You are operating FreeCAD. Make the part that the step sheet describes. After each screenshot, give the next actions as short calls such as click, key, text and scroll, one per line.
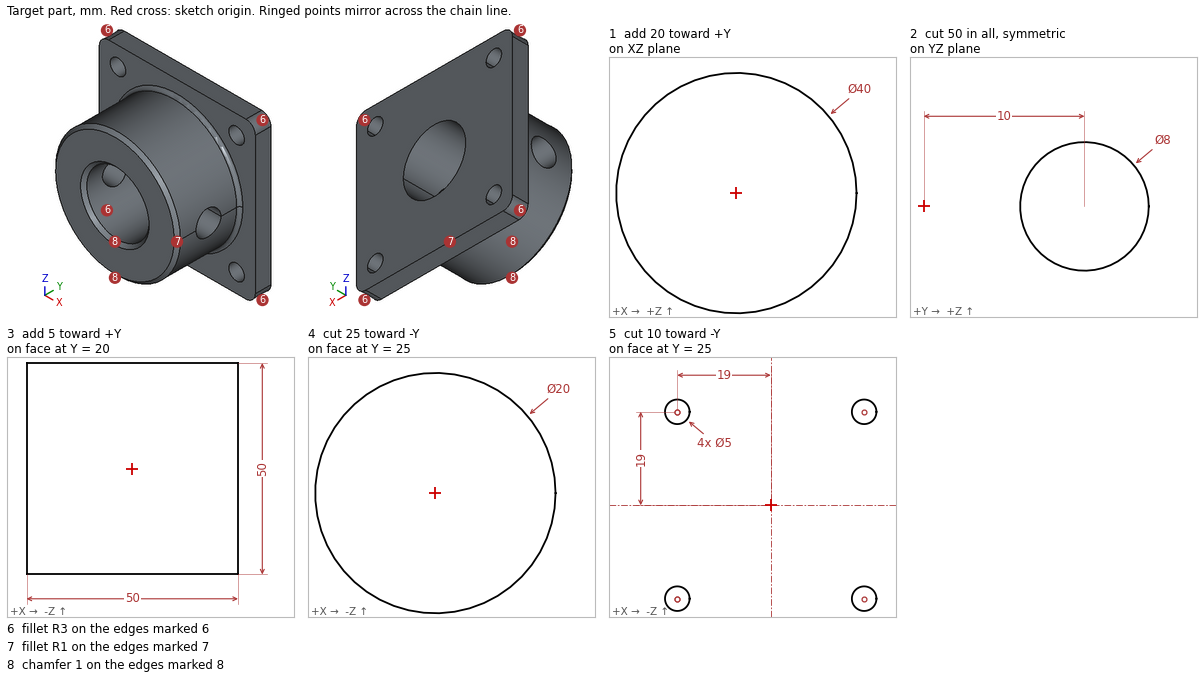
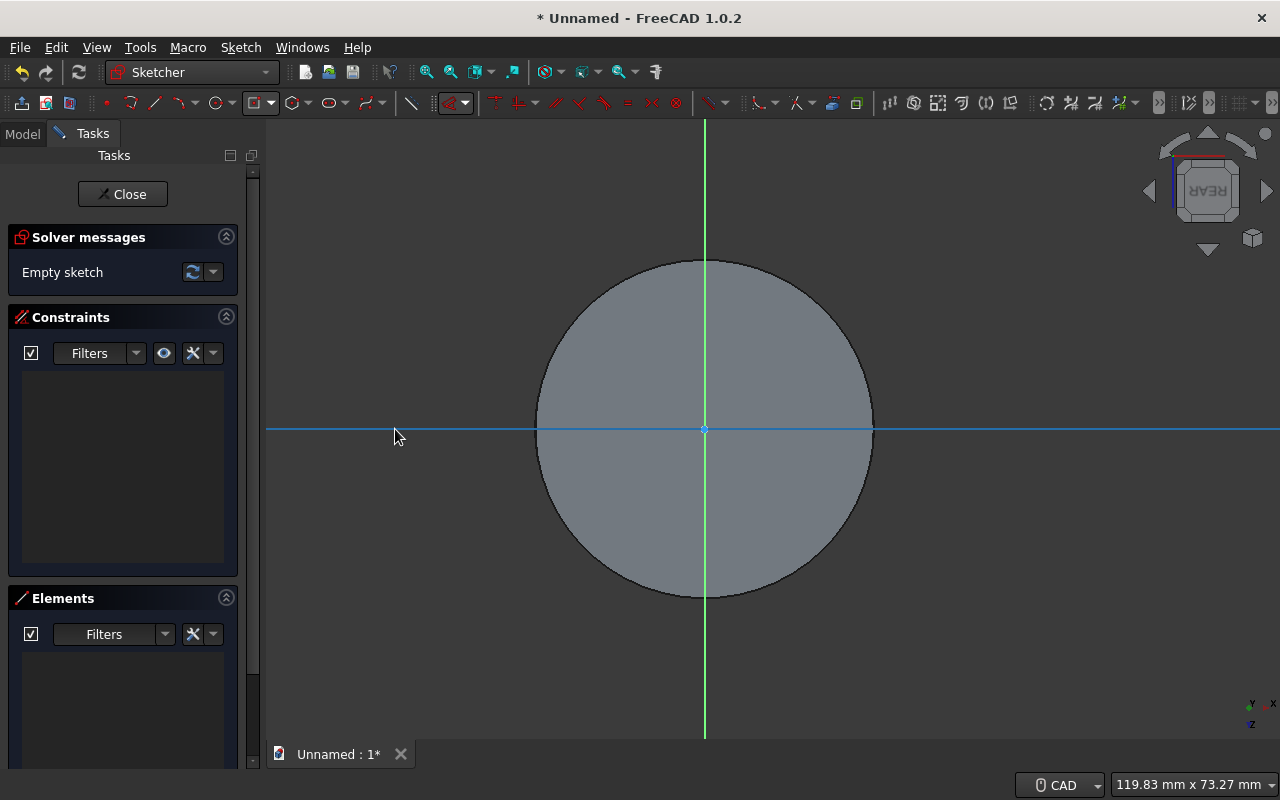
click(254, 104)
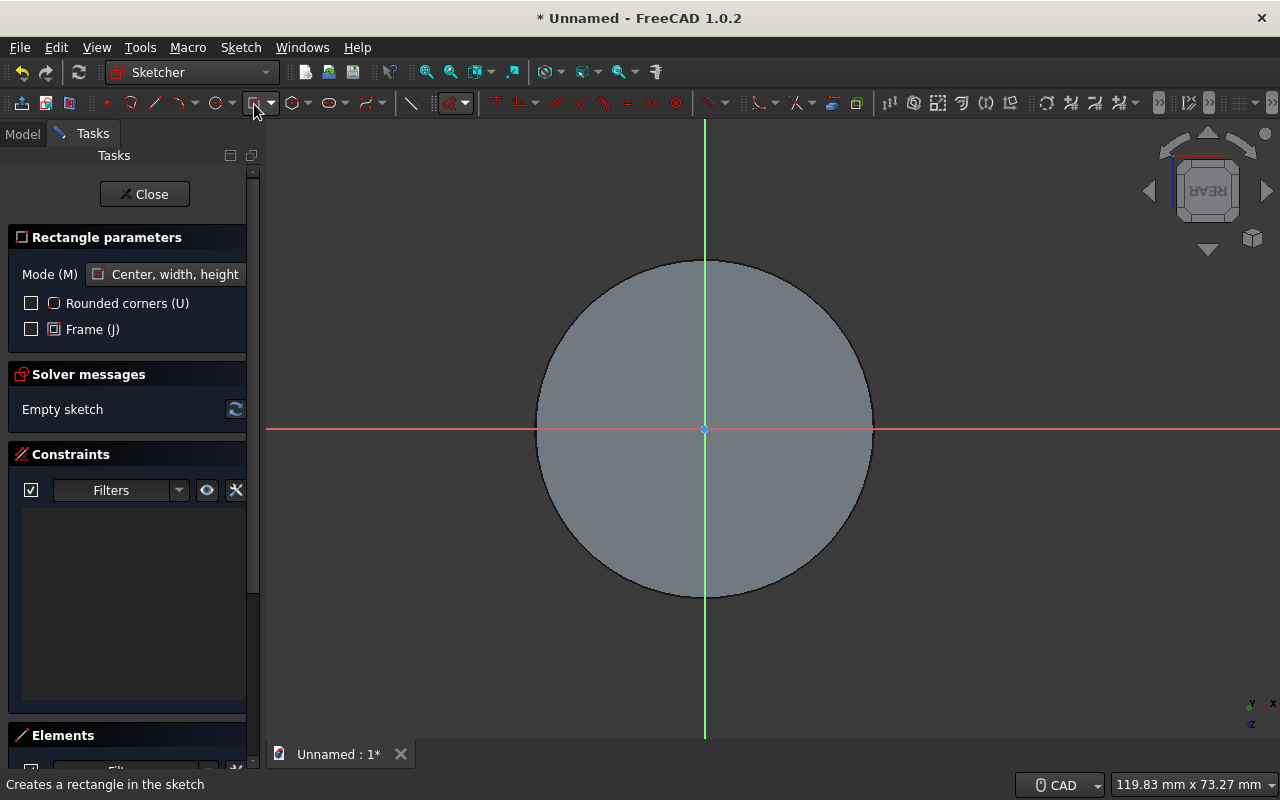
click(705, 429)
click(916, 218)
key(Escape)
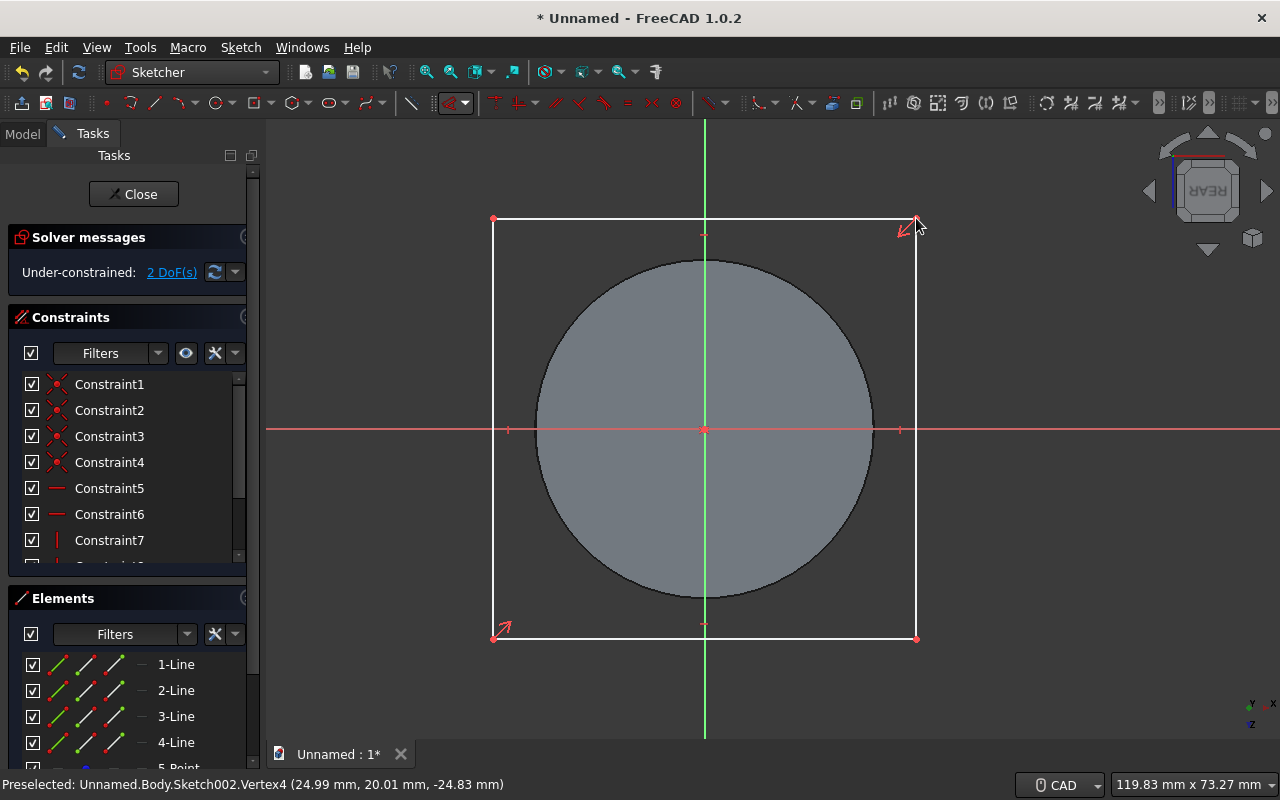
click(620, 639)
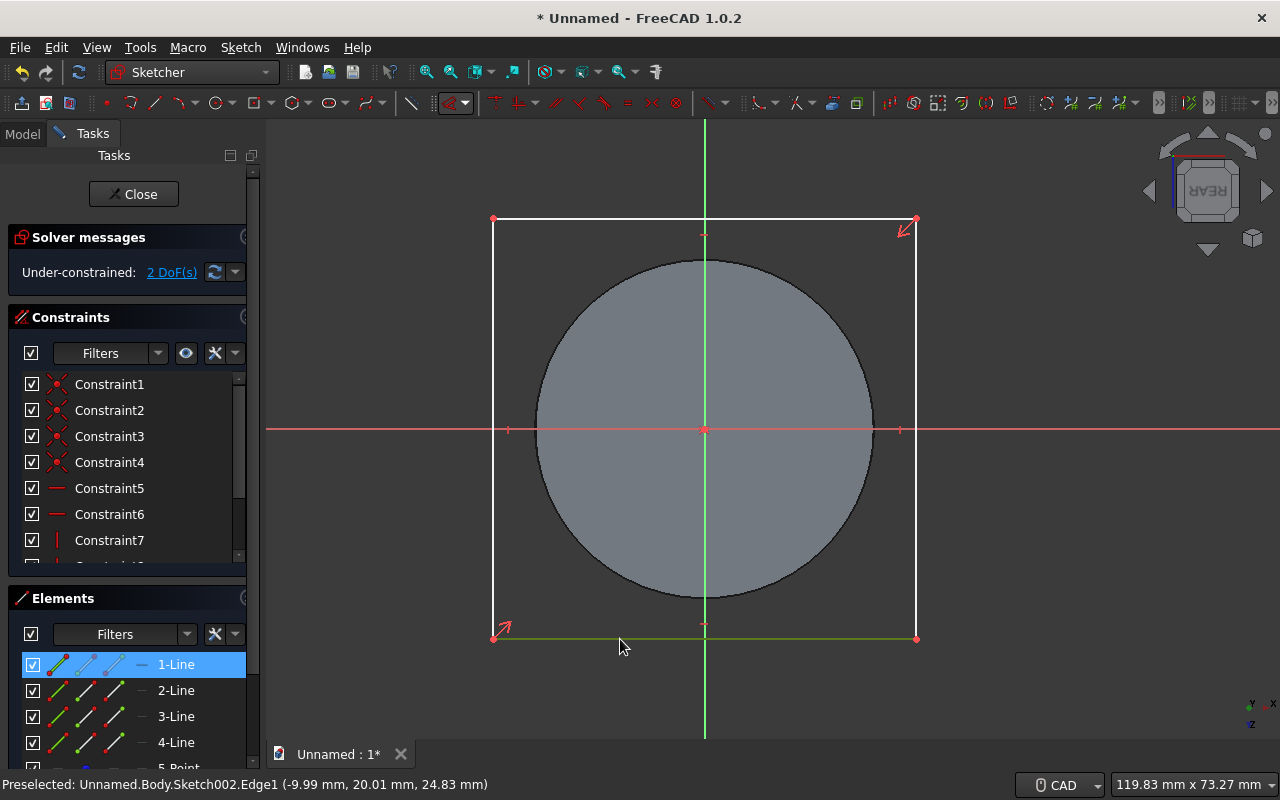
key(l)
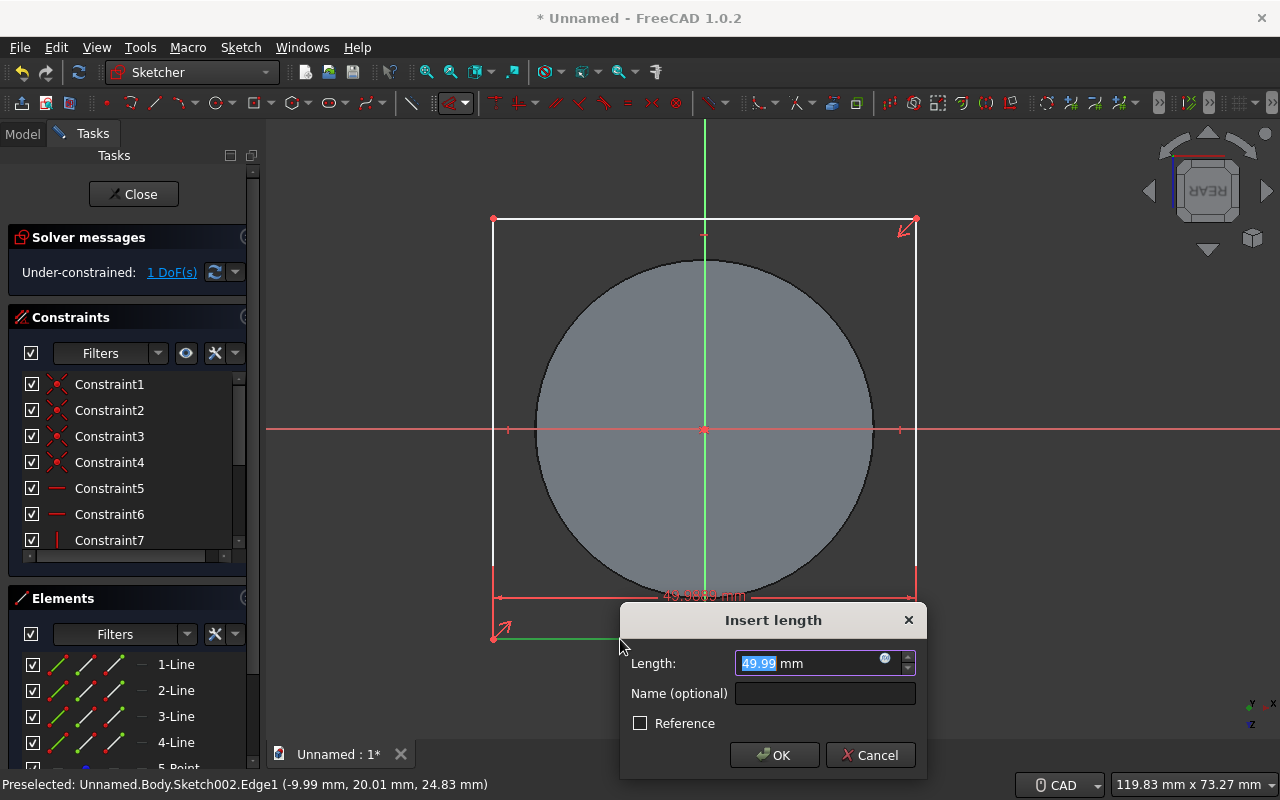
text(50)
key(Return)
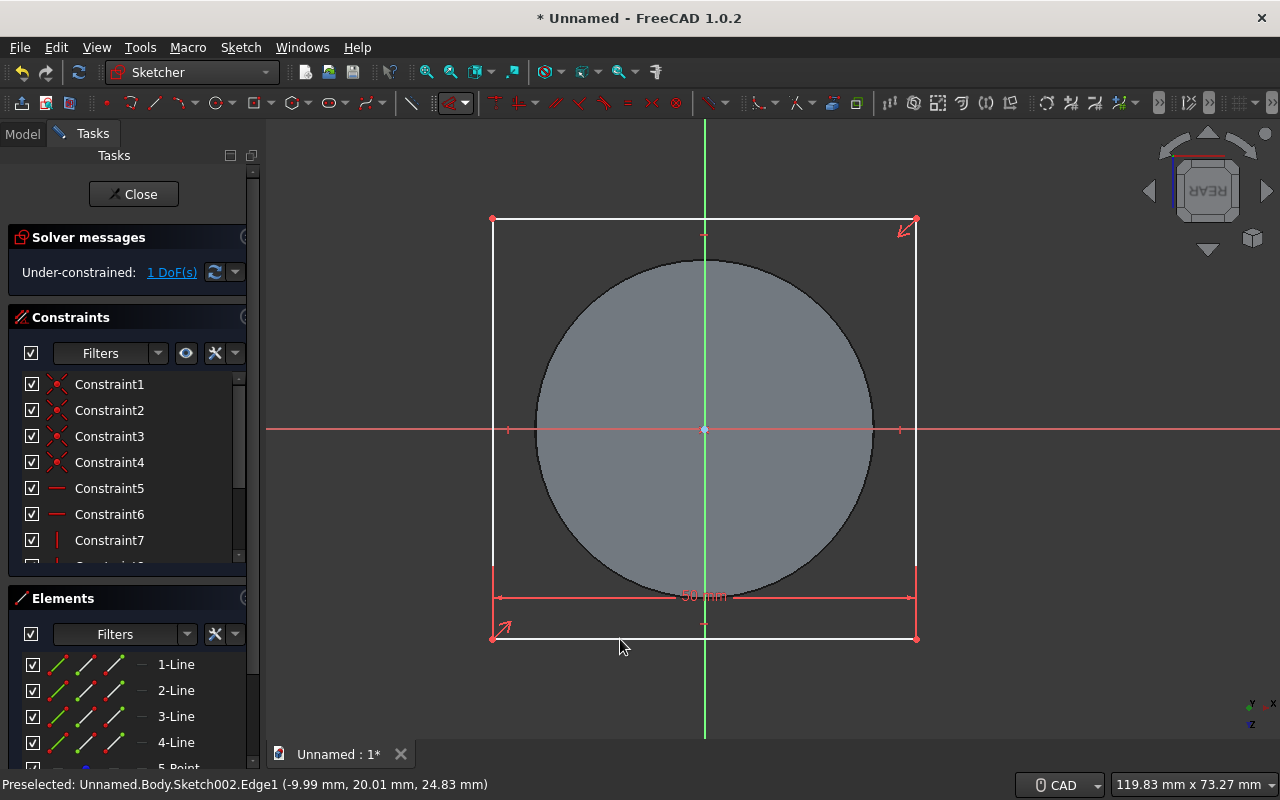
click(916, 513)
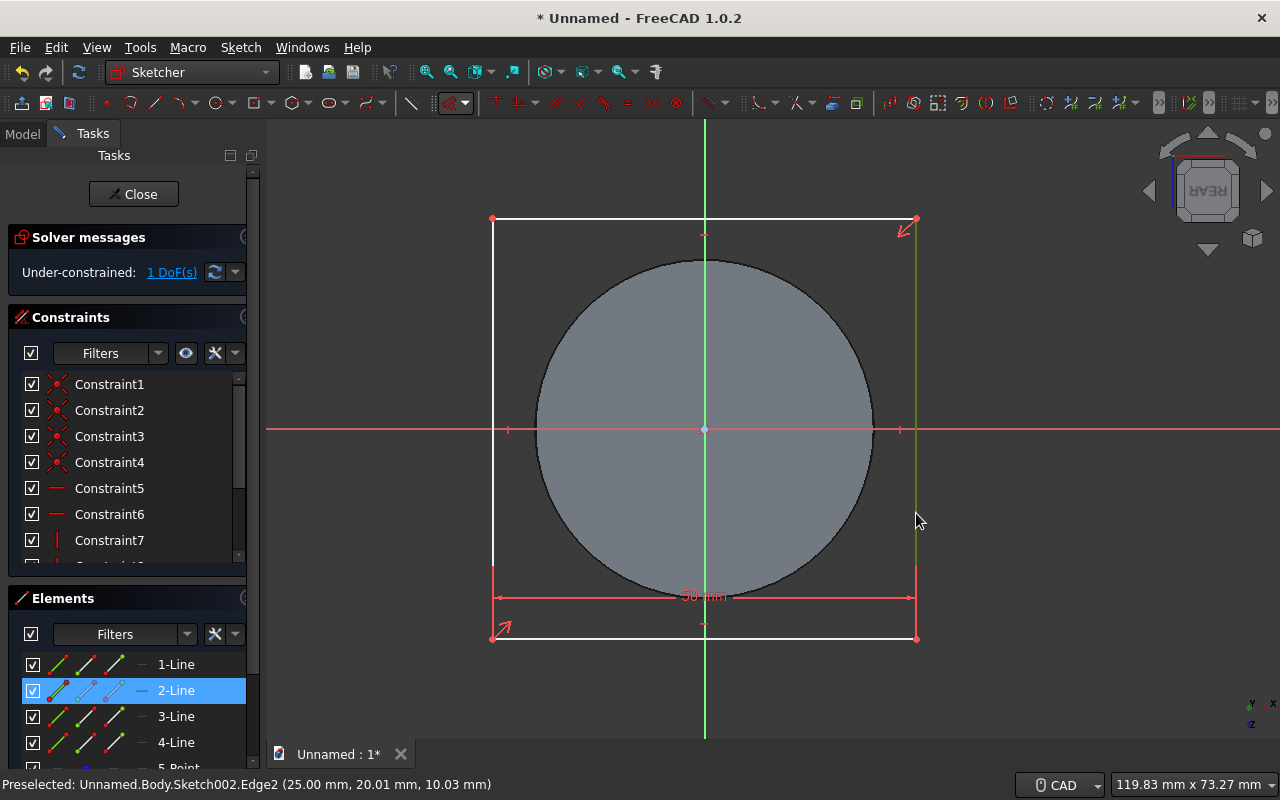
key(i)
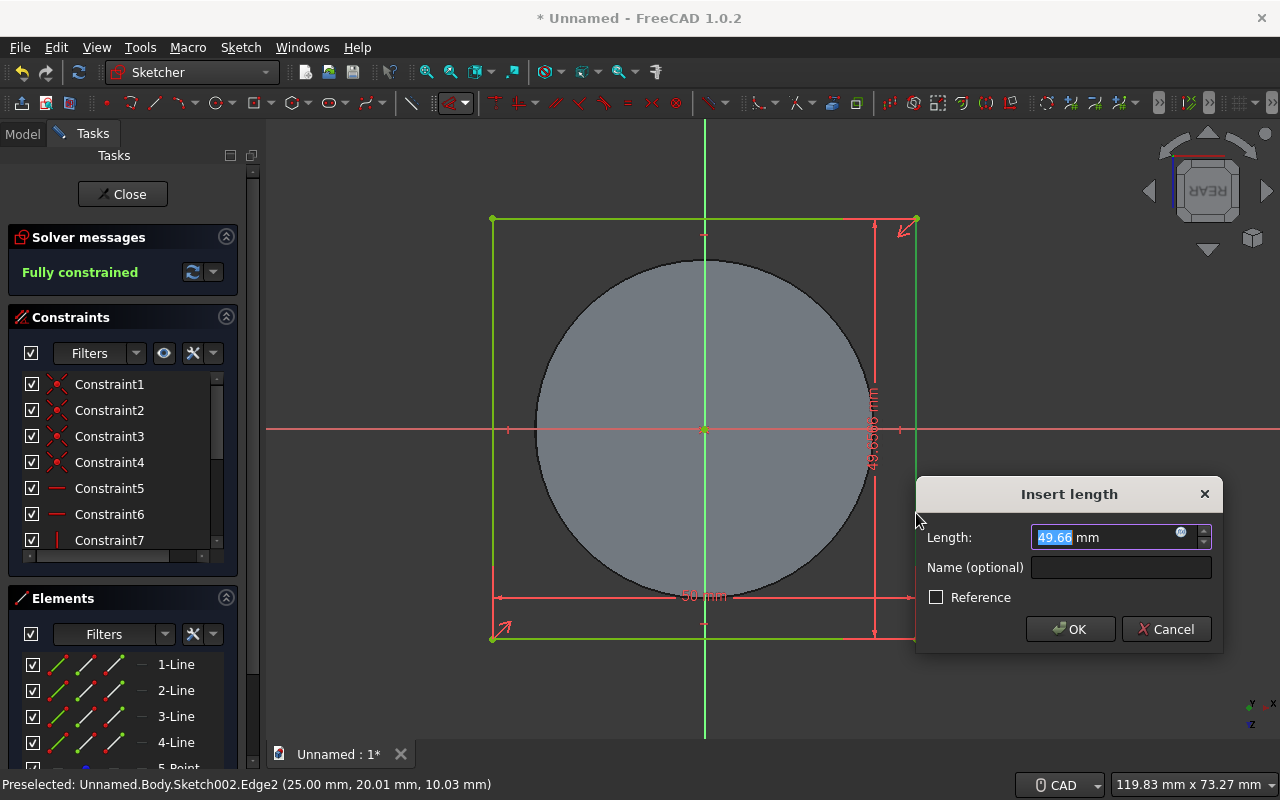
text(50)
key(Return)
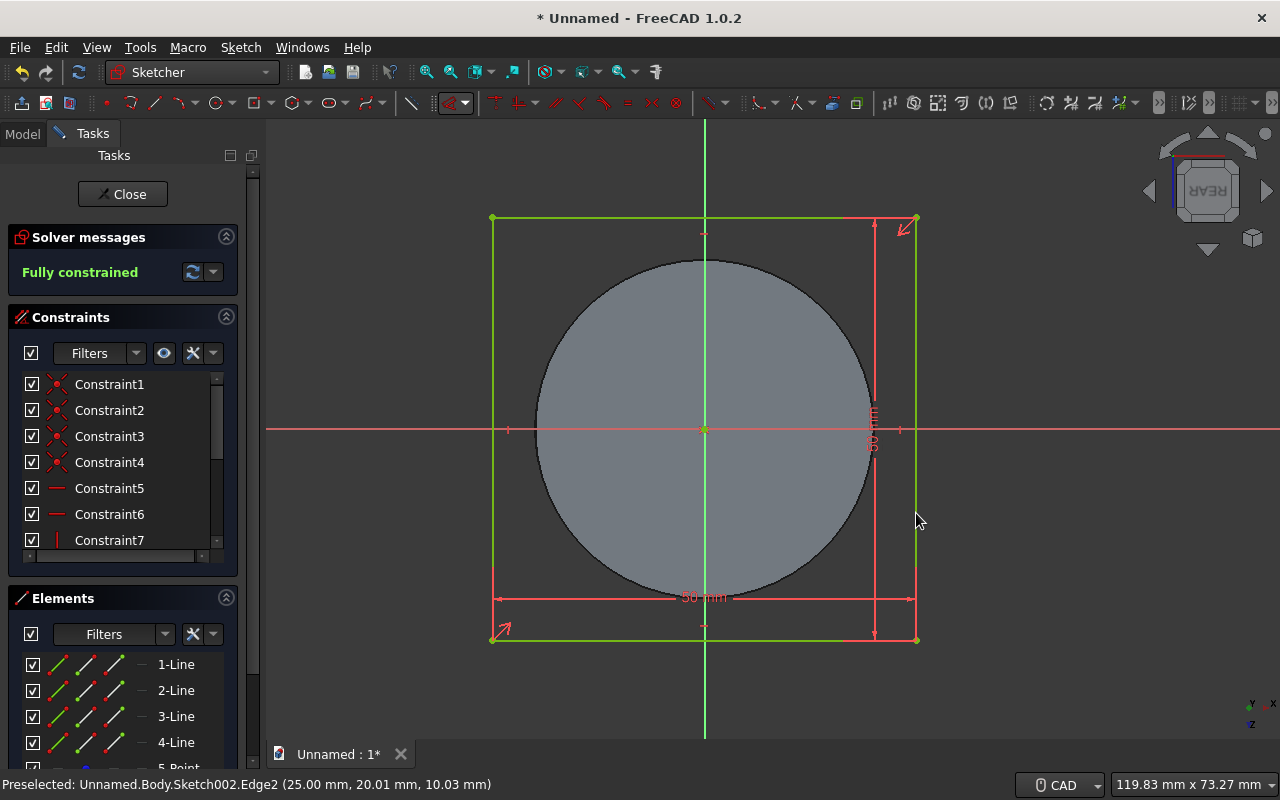
click(123, 194)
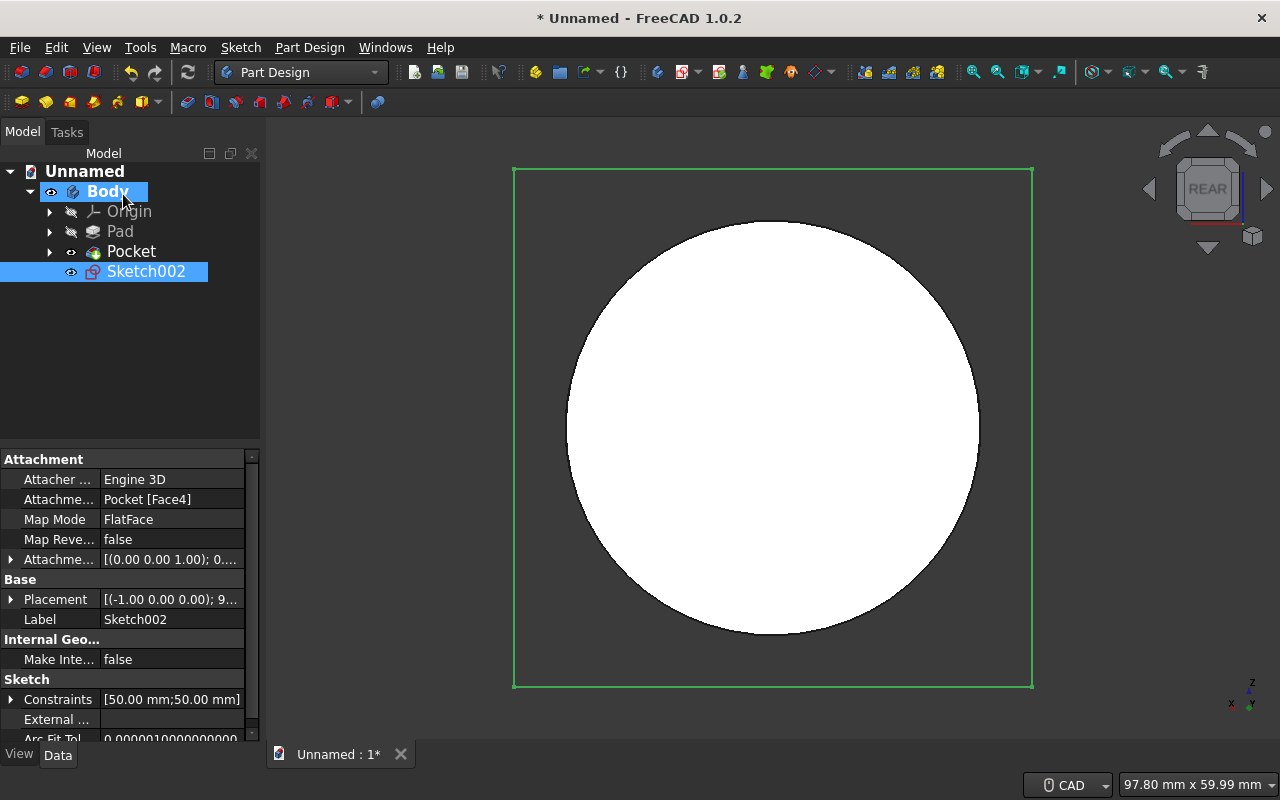
click(22, 102)